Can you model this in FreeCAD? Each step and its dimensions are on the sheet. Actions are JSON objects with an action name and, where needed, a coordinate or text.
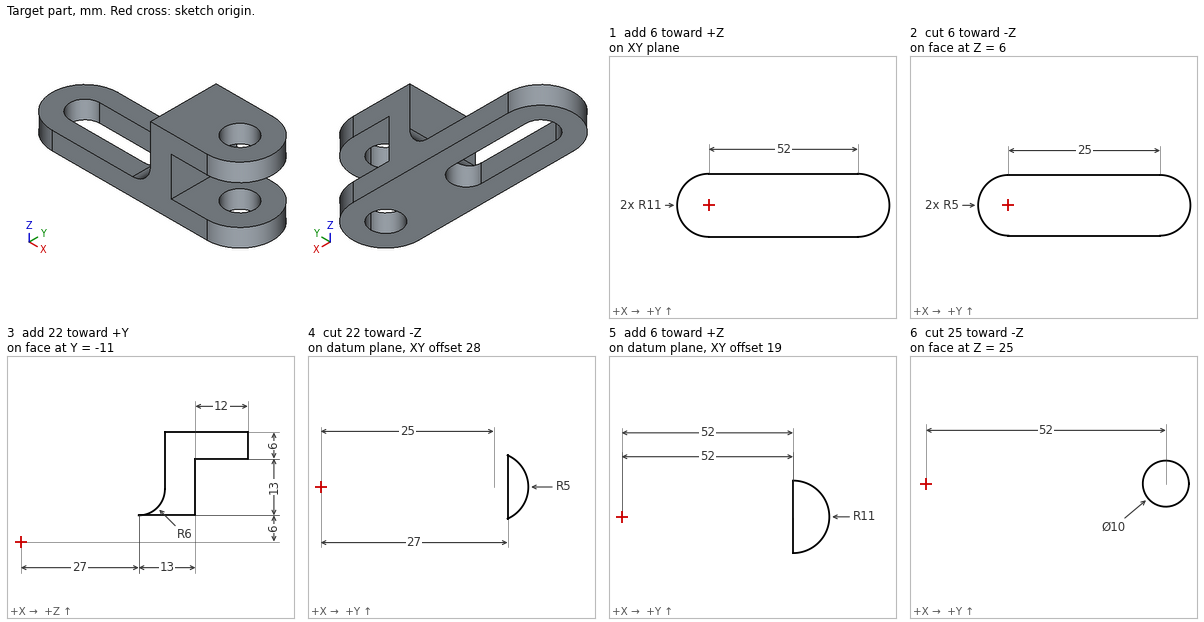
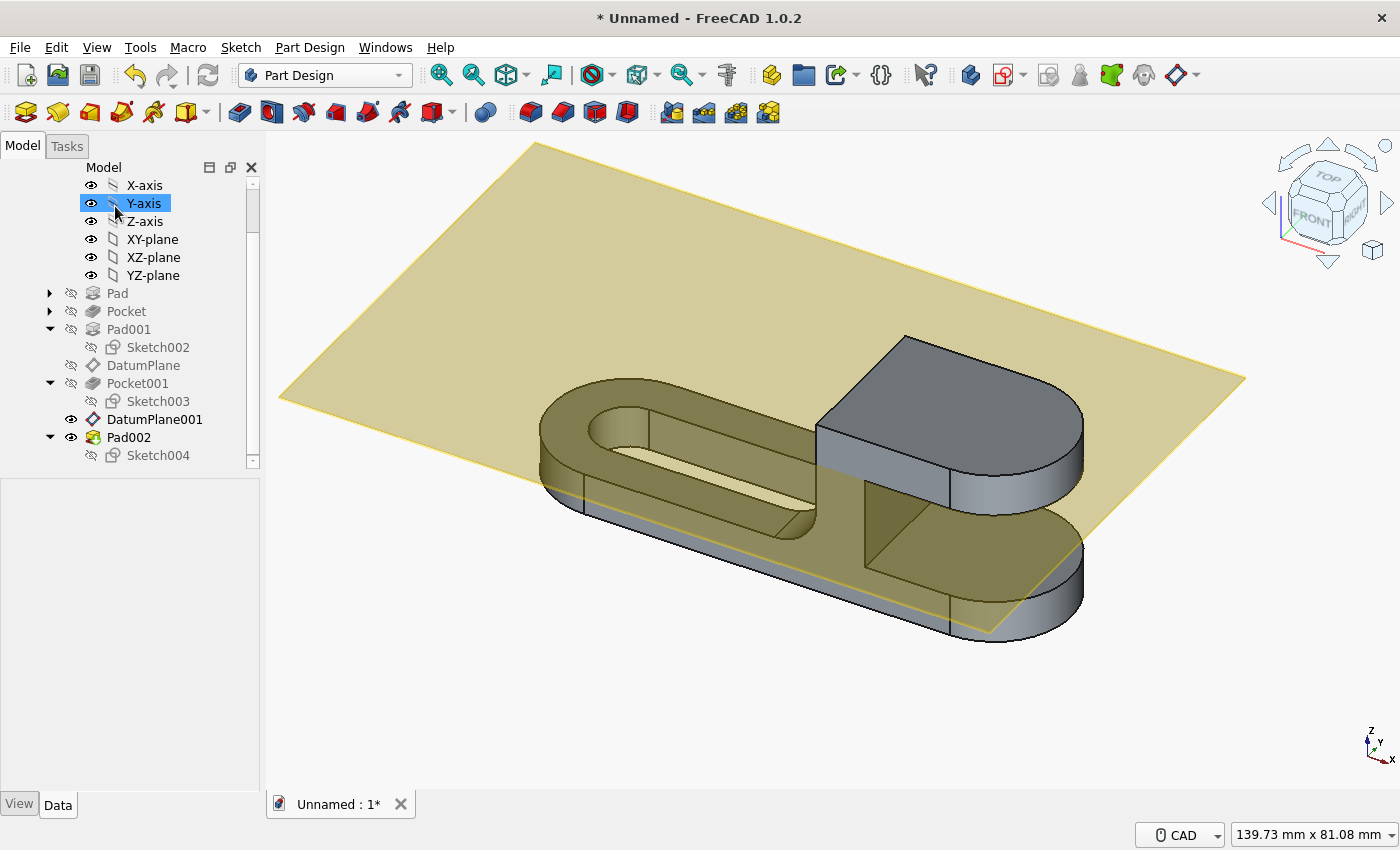
{"action": "left_click", "coordinate": [116, 419]}
{"action": "key", "text": "space"}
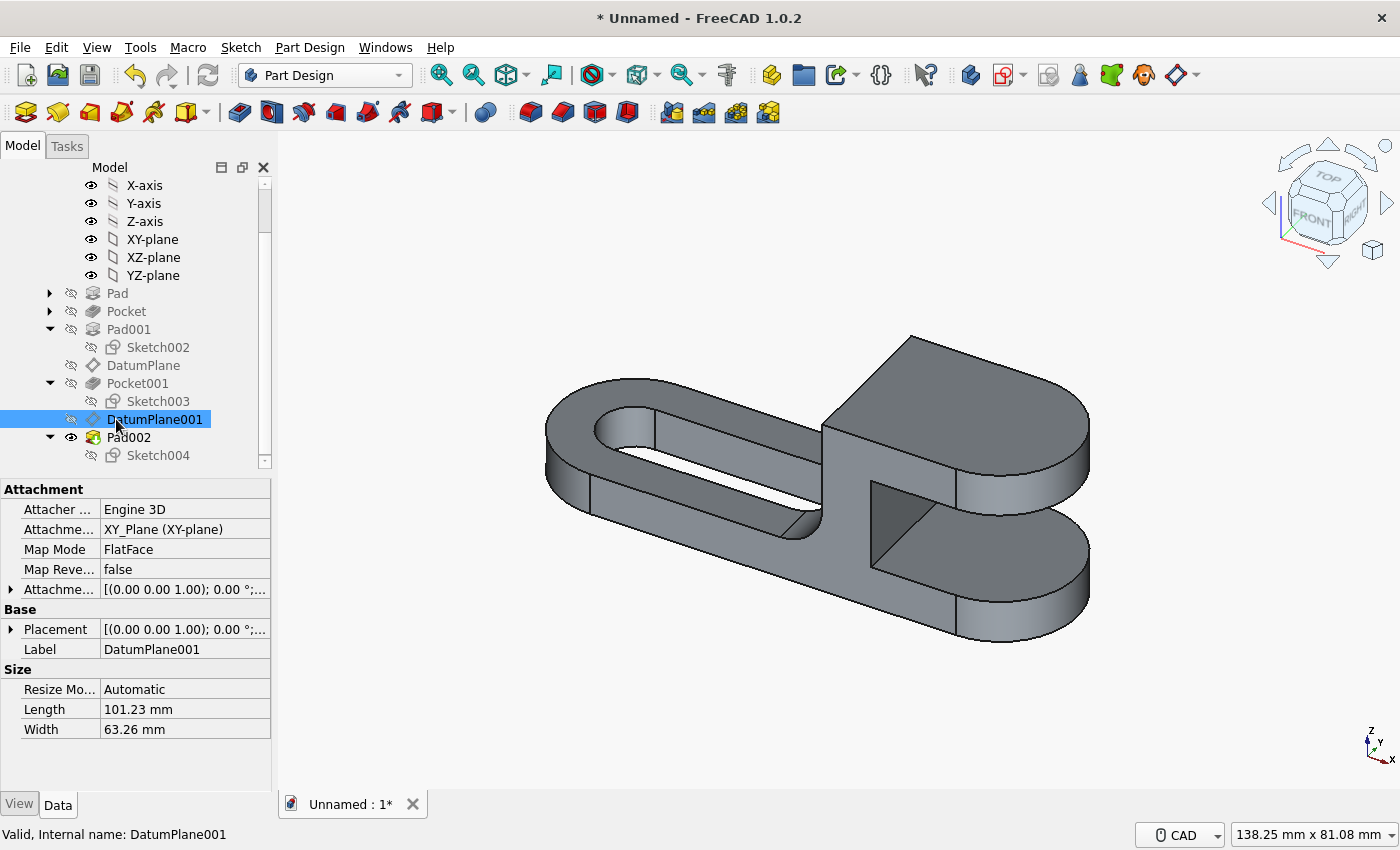
{"action": "left_click", "coordinate": [972, 414]}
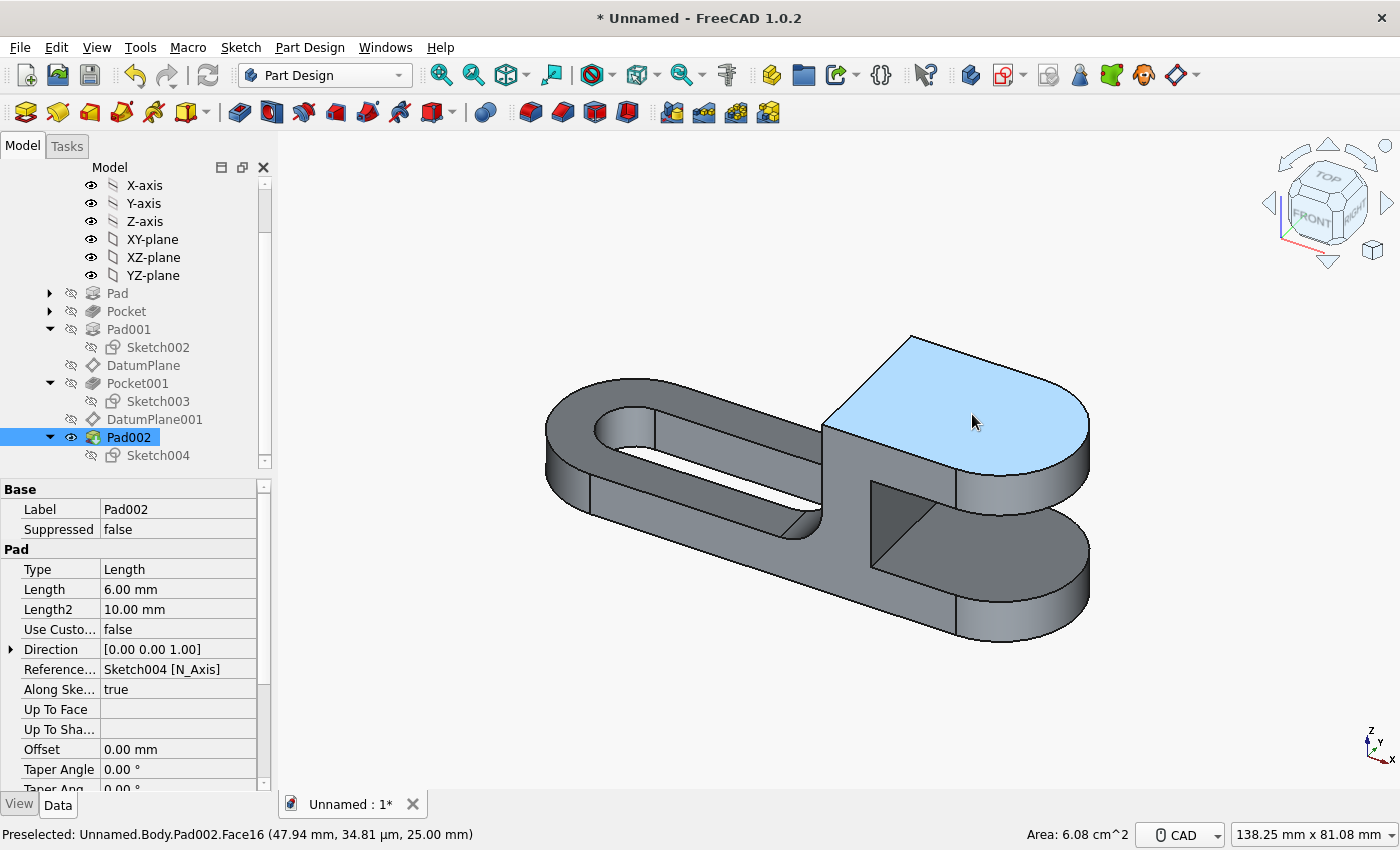
{"action": "left_click", "coordinate": [1004, 76]}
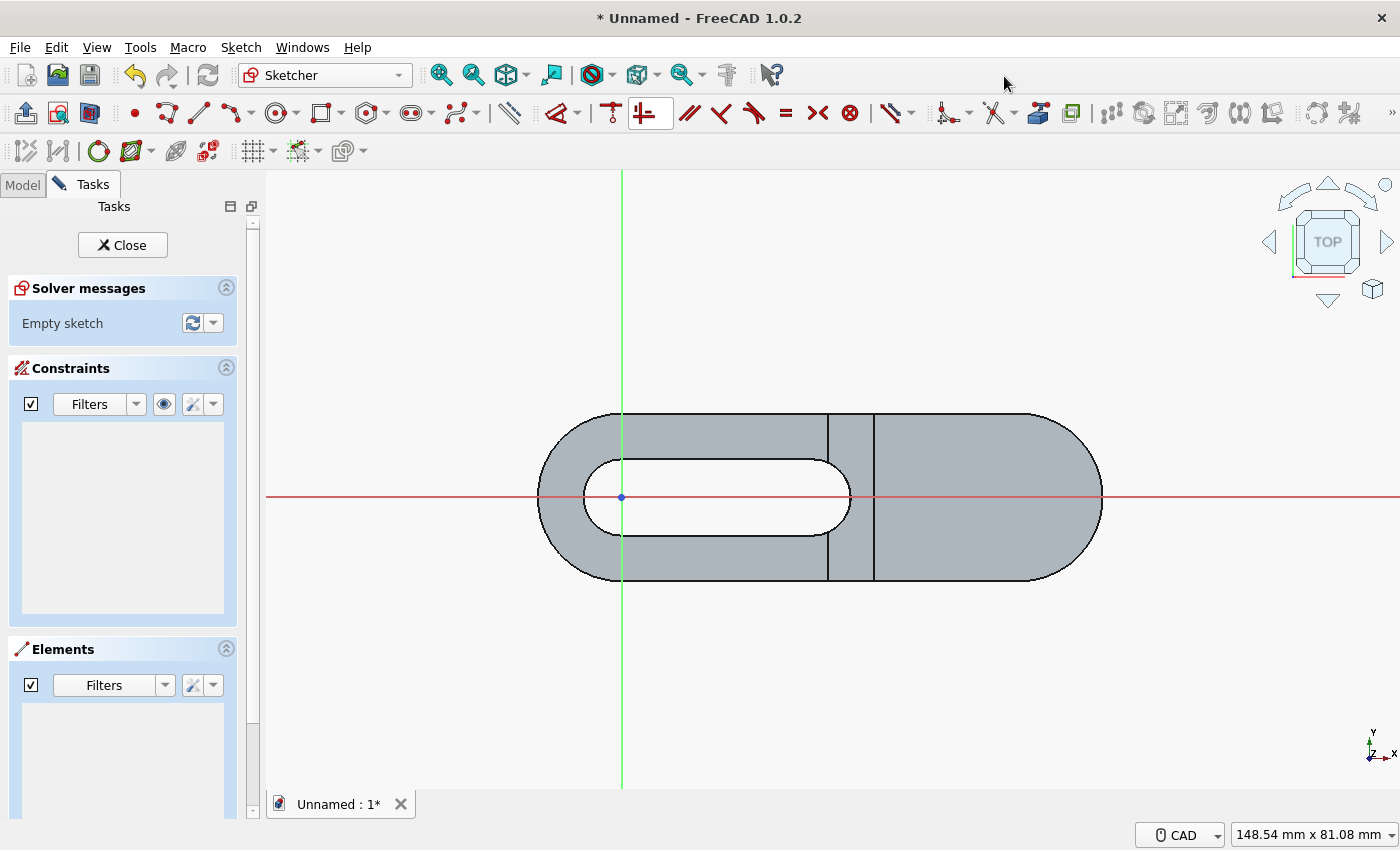
{"action": "scroll", "coordinate": [1083, 502], "scroll_direction": "up", "scroll_amount": 8}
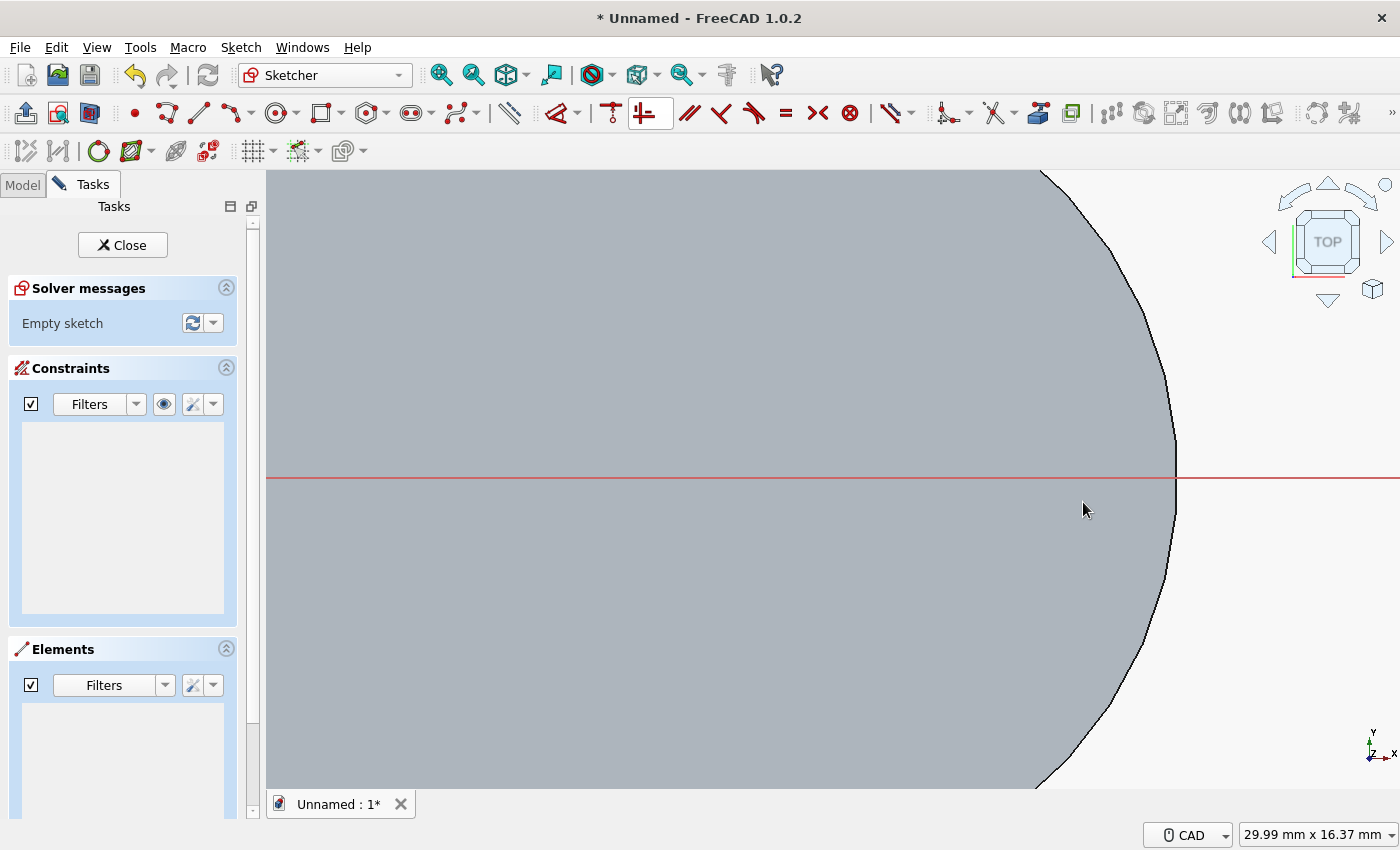
{"action": "left_click", "coordinate": [276, 114]}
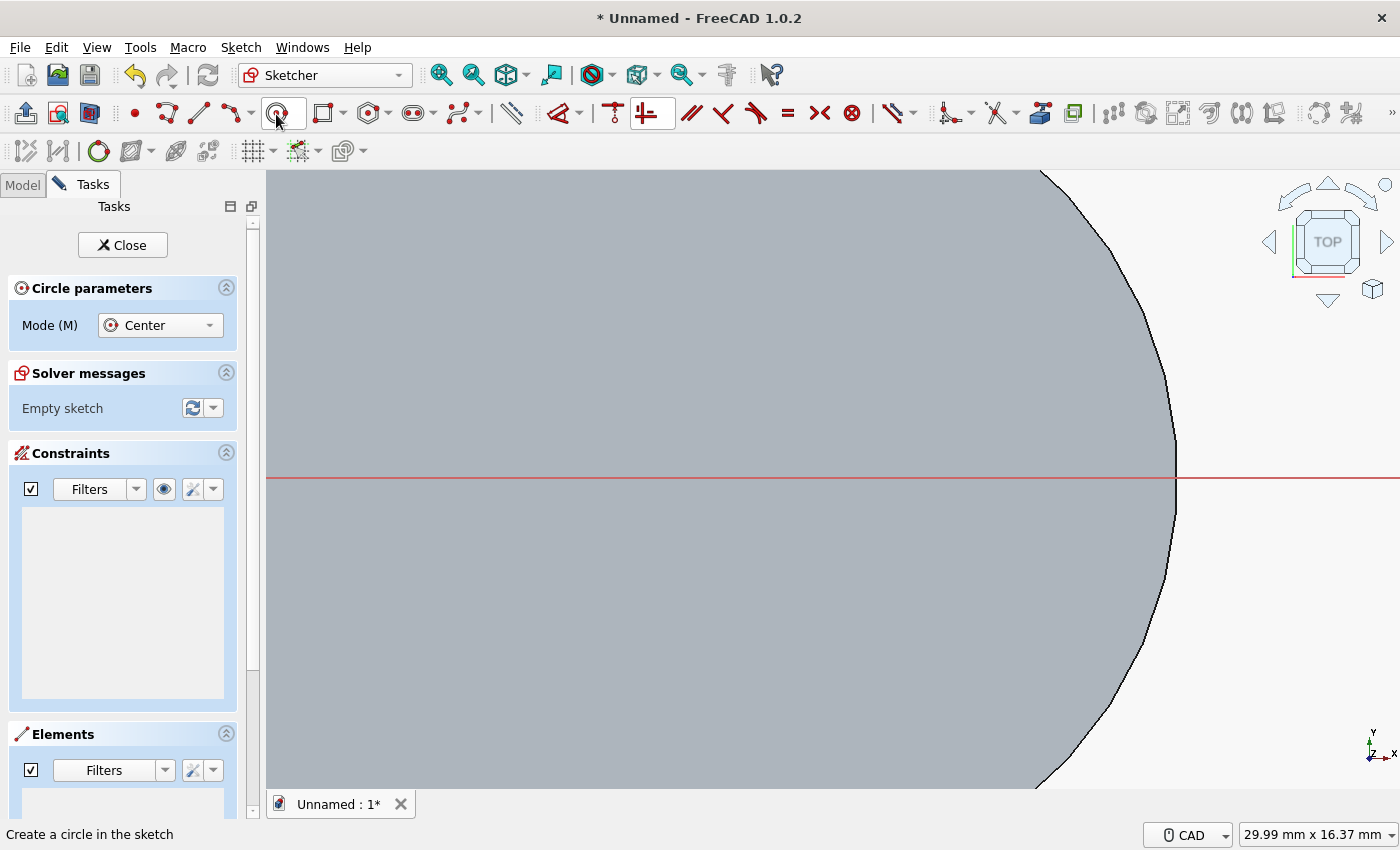
{"action": "left_click", "coordinate": [762, 478]}
{"action": "left_click", "coordinate": [895, 344]}
{"action": "key", "text": "Escape"}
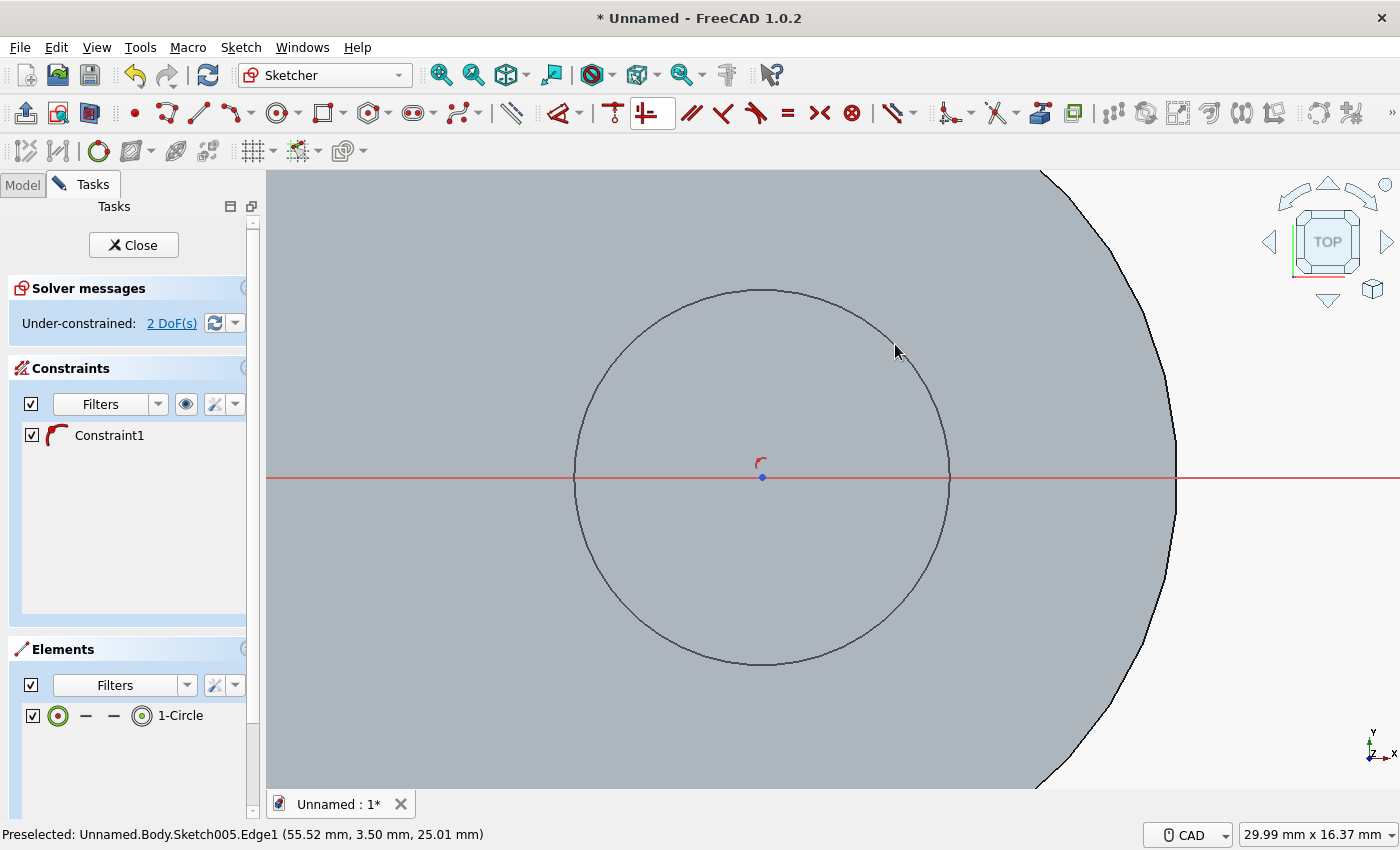
{"action": "left_click", "coordinate": [558, 114]}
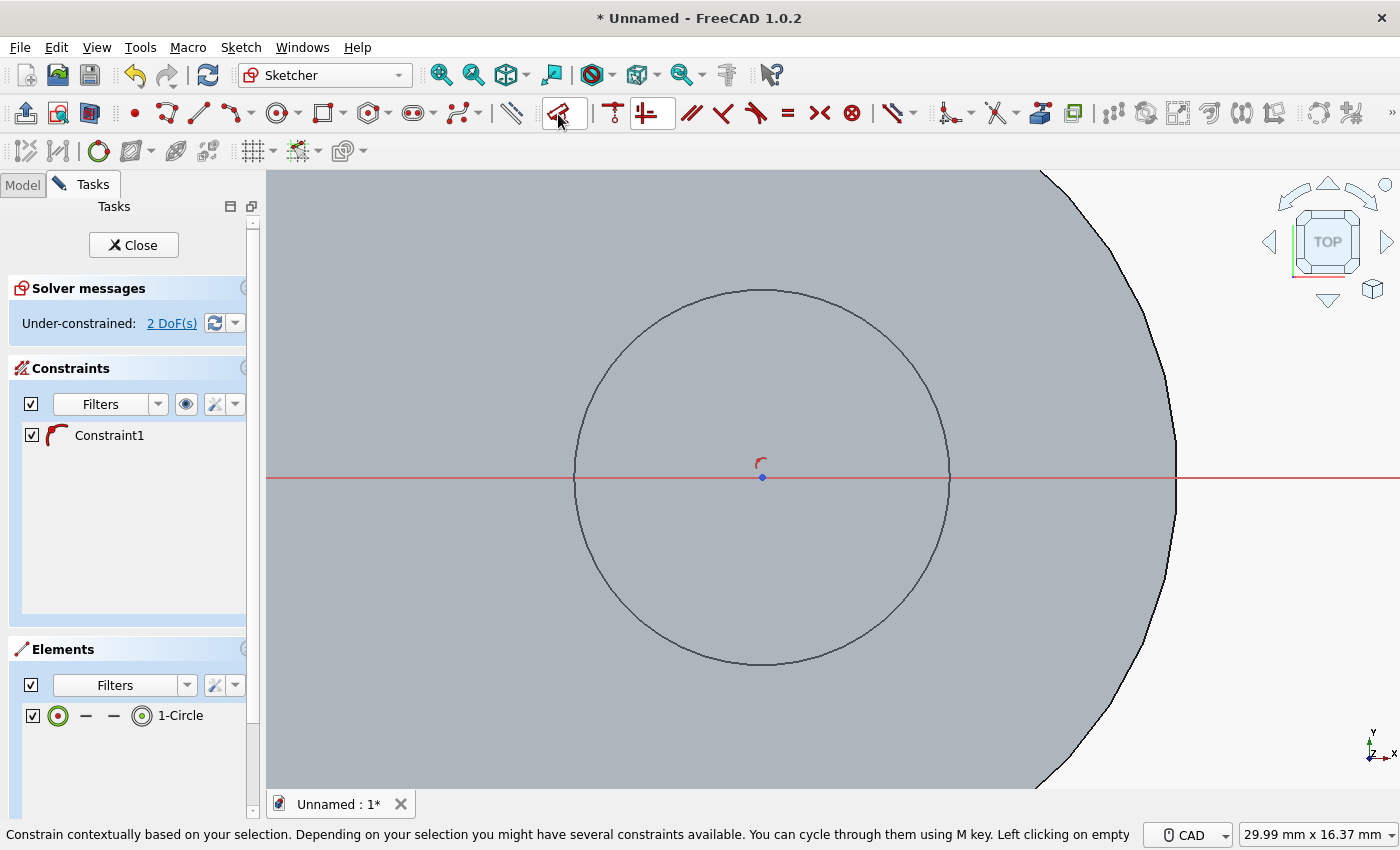
{"action": "left_click", "coordinate": [894, 344]}
{"action": "left_click", "coordinate": [916, 321]}